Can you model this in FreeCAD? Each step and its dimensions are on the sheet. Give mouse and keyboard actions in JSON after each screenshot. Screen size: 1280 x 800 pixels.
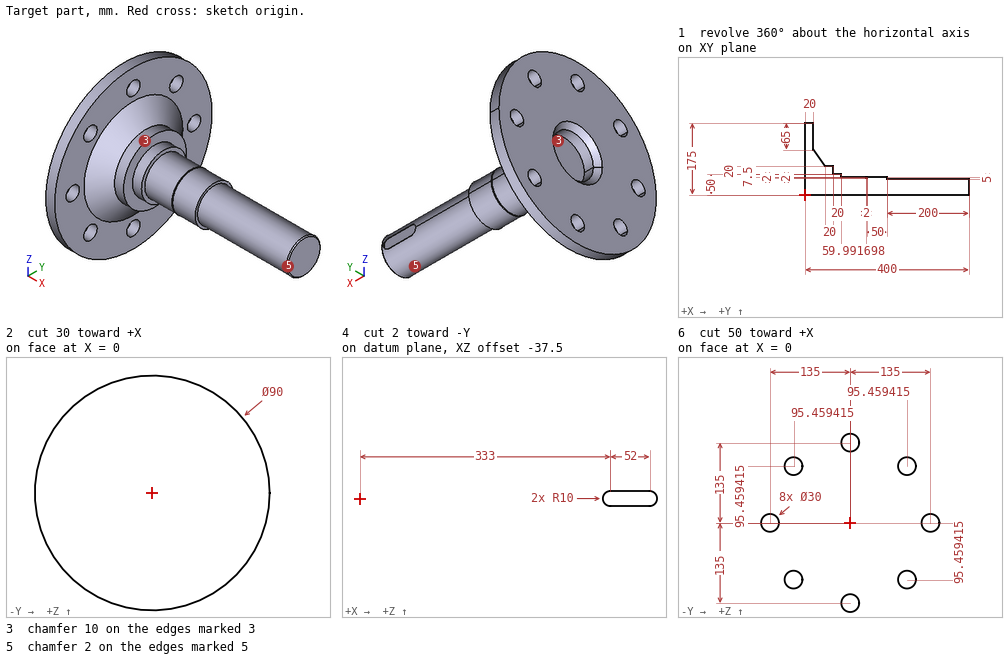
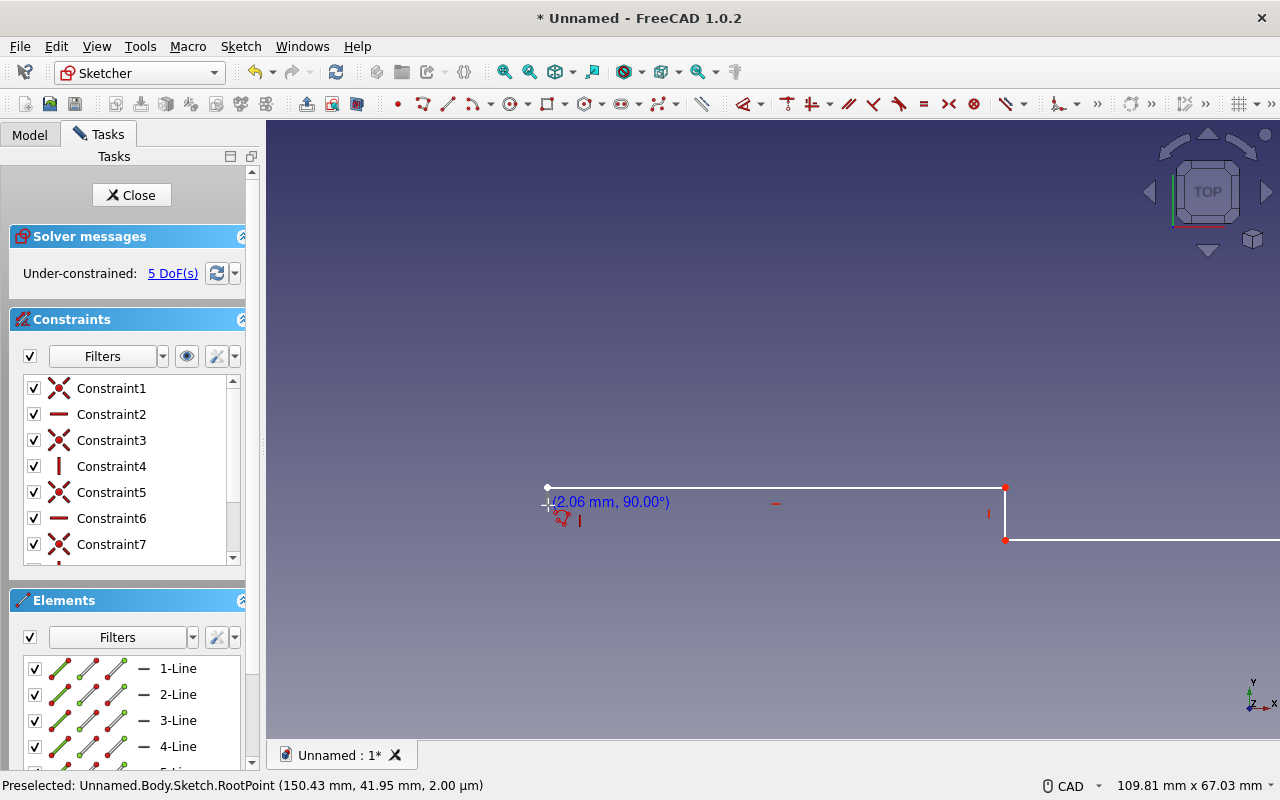
{"action": "left_click", "coordinate": [548, 504]}
{"action": "left_click", "coordinate": [528, 504]}
{"action": "left_click", "coordinate": [528, 485]}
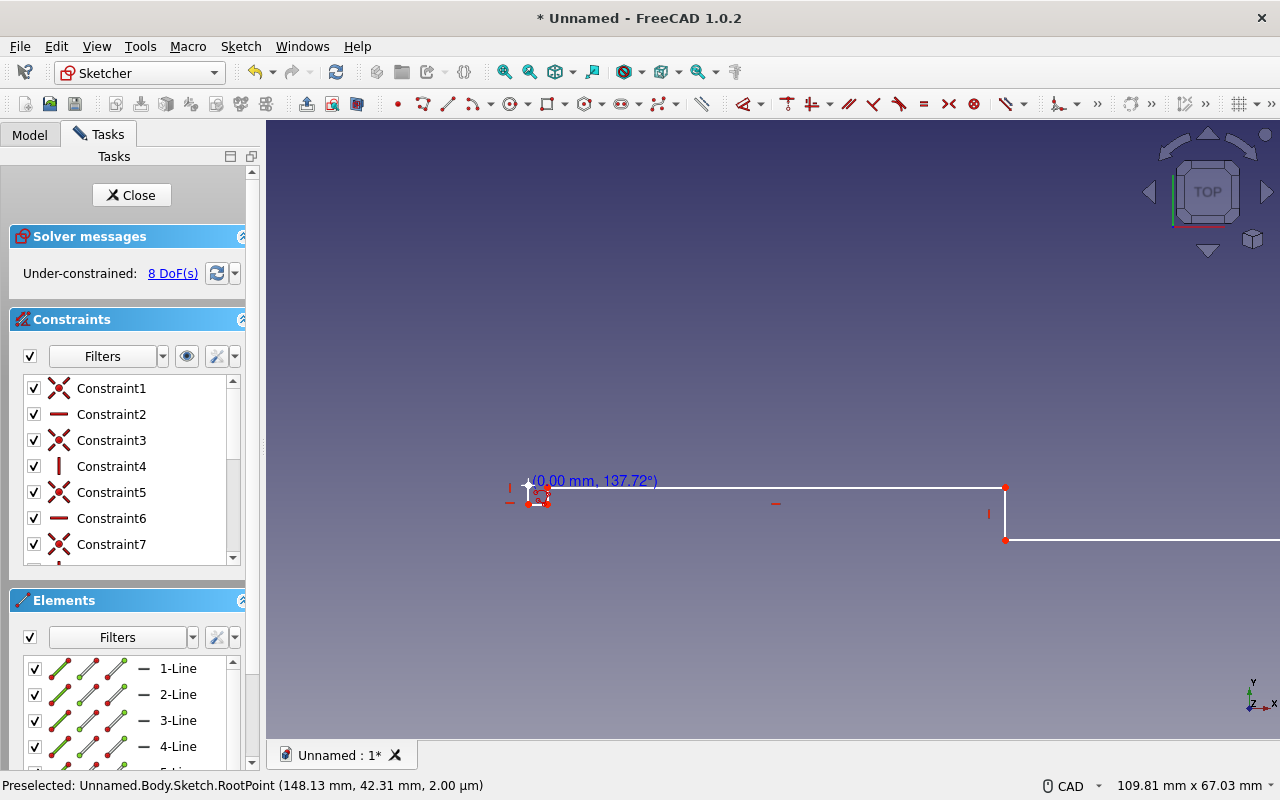
{"action": "scroll", "coordinate": [644, 501], "scroll_direction": "down", "scroll_amount": 9}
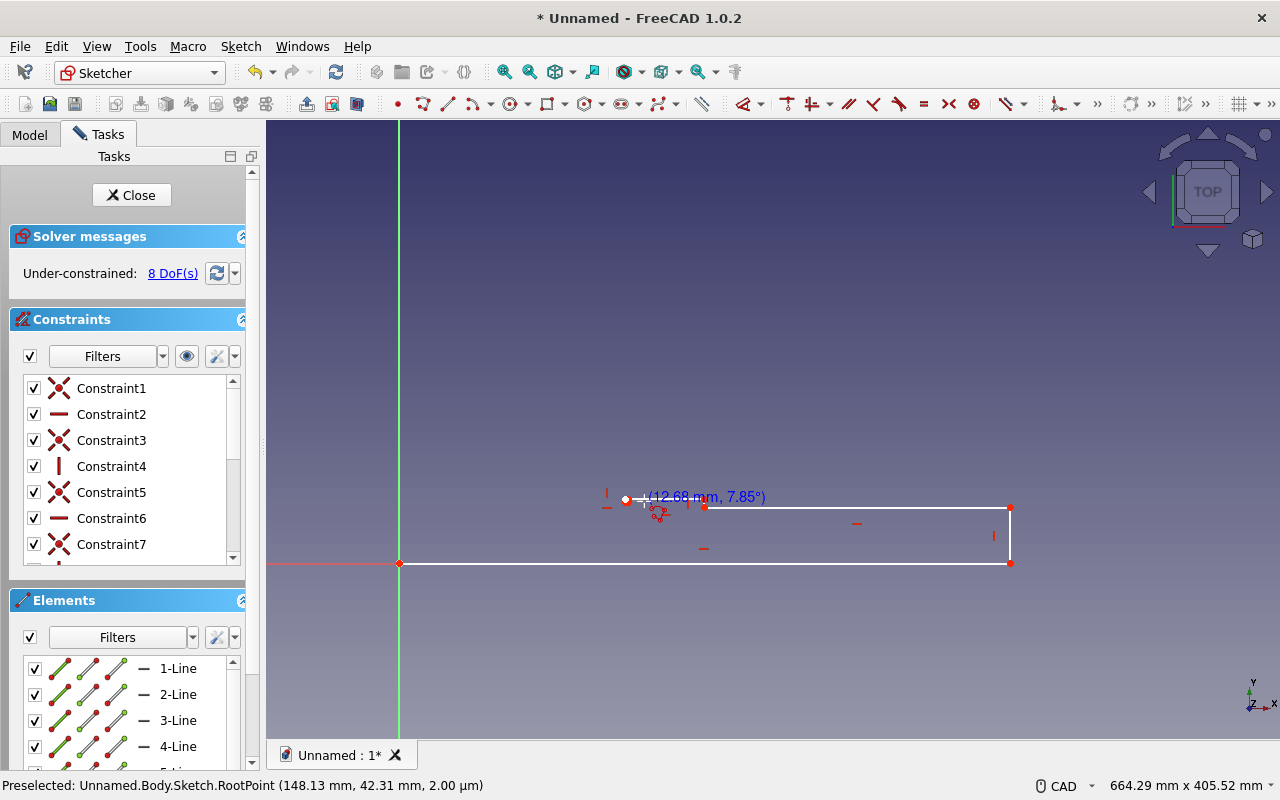
{"action": "left_click", "coordinate": [534, 499]}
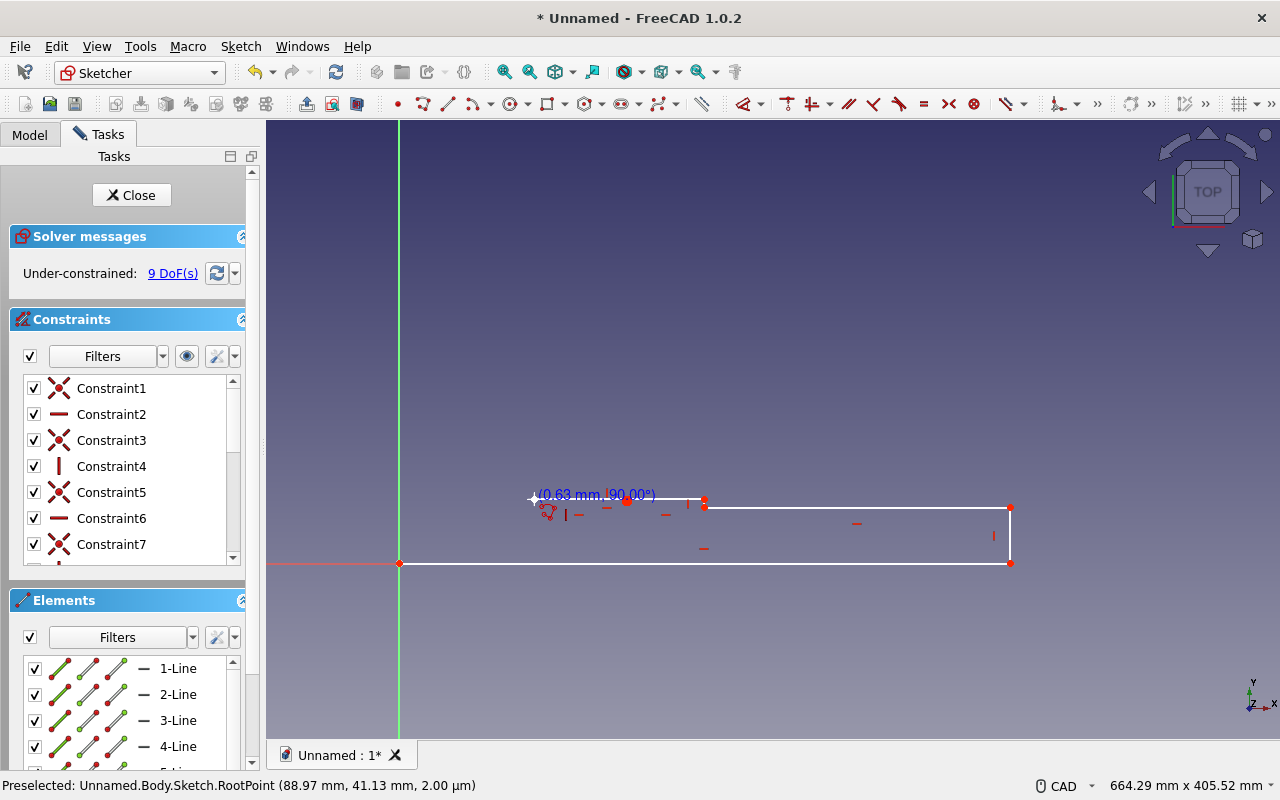
{"action": "scroll", "coordinate": [534, 487], "scroll_direction": "up", "scroll_amount": 2}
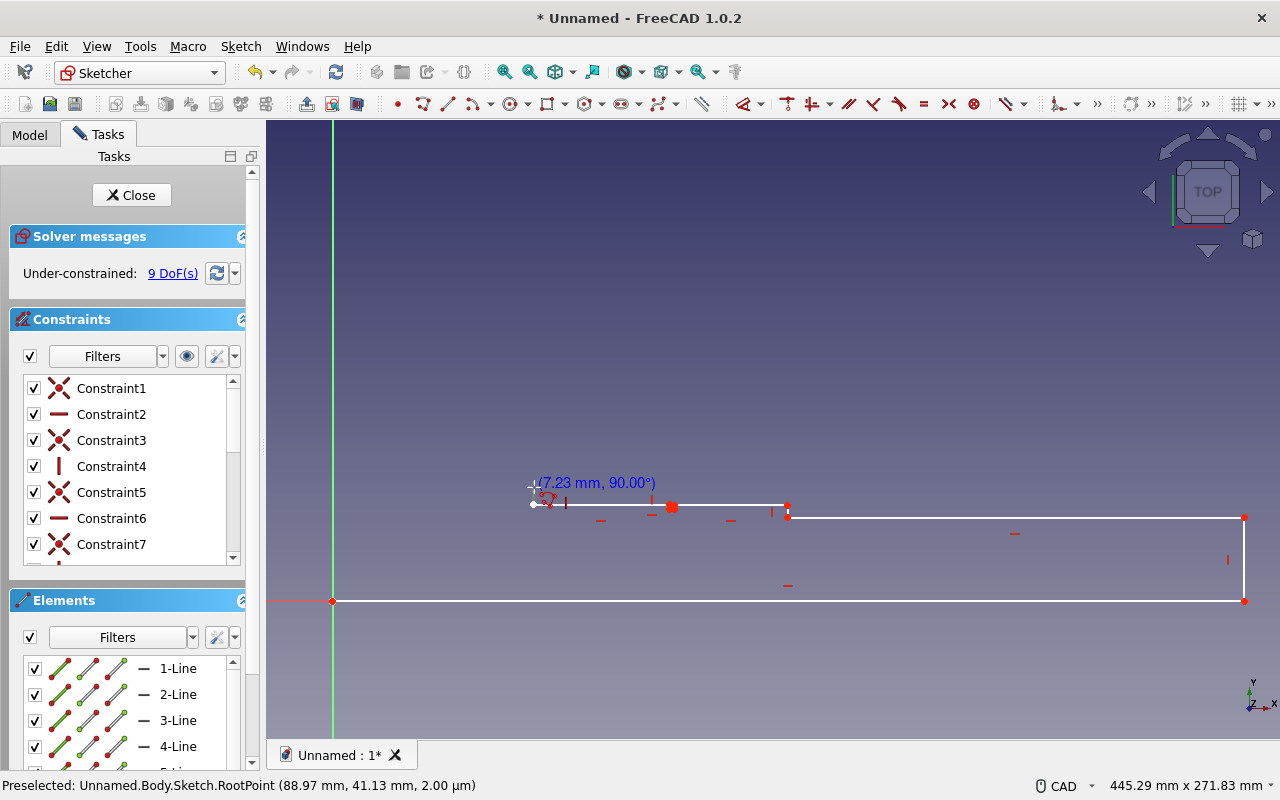
{"action": "left_click", "coordinate": [534, 487]}
{"action": "left_click", "coordinate": [488, 487]}
{"action": "left_click", "coordinate": [488, 442]}
{"action": "left_click", "coordinate": [442, 442]}
{"action": "left_click", "coordinate": [378, 351]}
{"action": "left_click", "coordinate": [378, 203]}
{"action": "left_click", "coordinate": [342, 203]}
{"action": "left_click", "coordinate": [333, 601]}
{"action": "key", "text": "Escape"}
{"action": "key", "text": "Escape"}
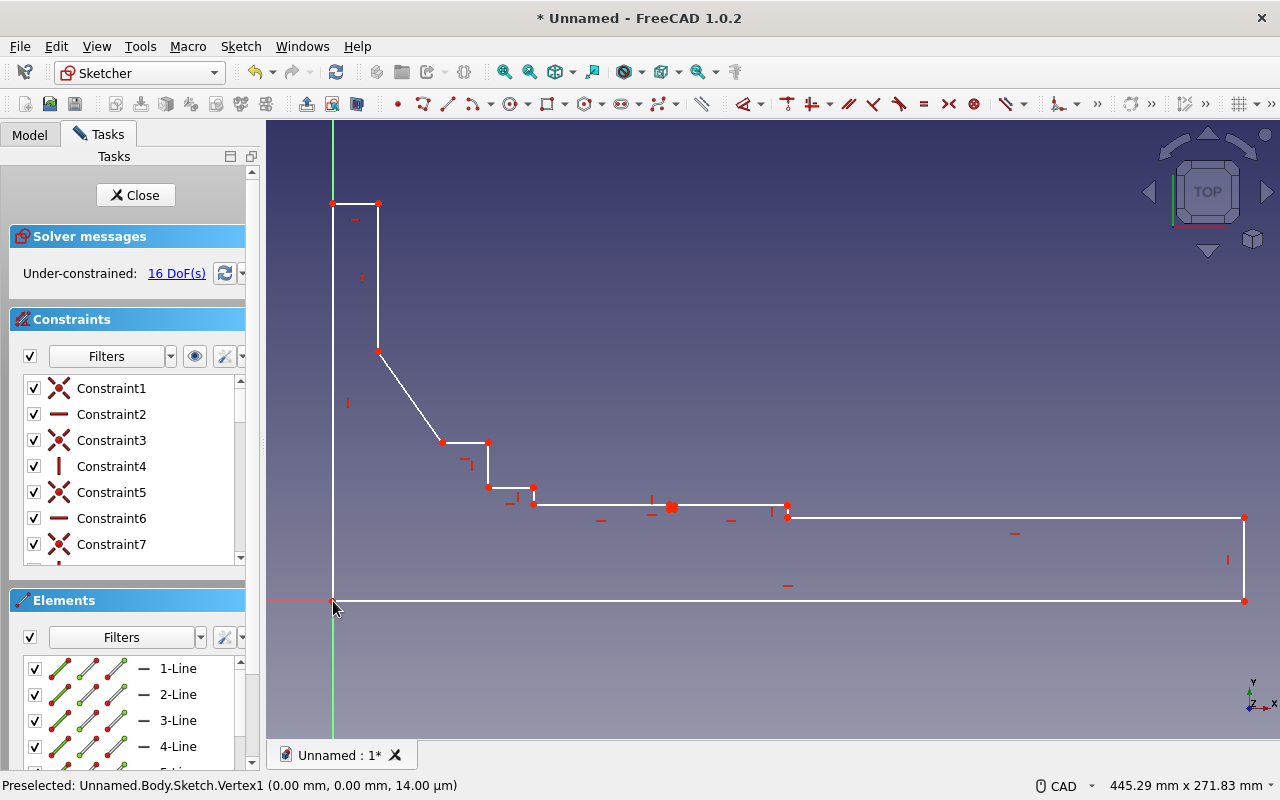
{"action": "left_click", "coordinate": [742, 104]}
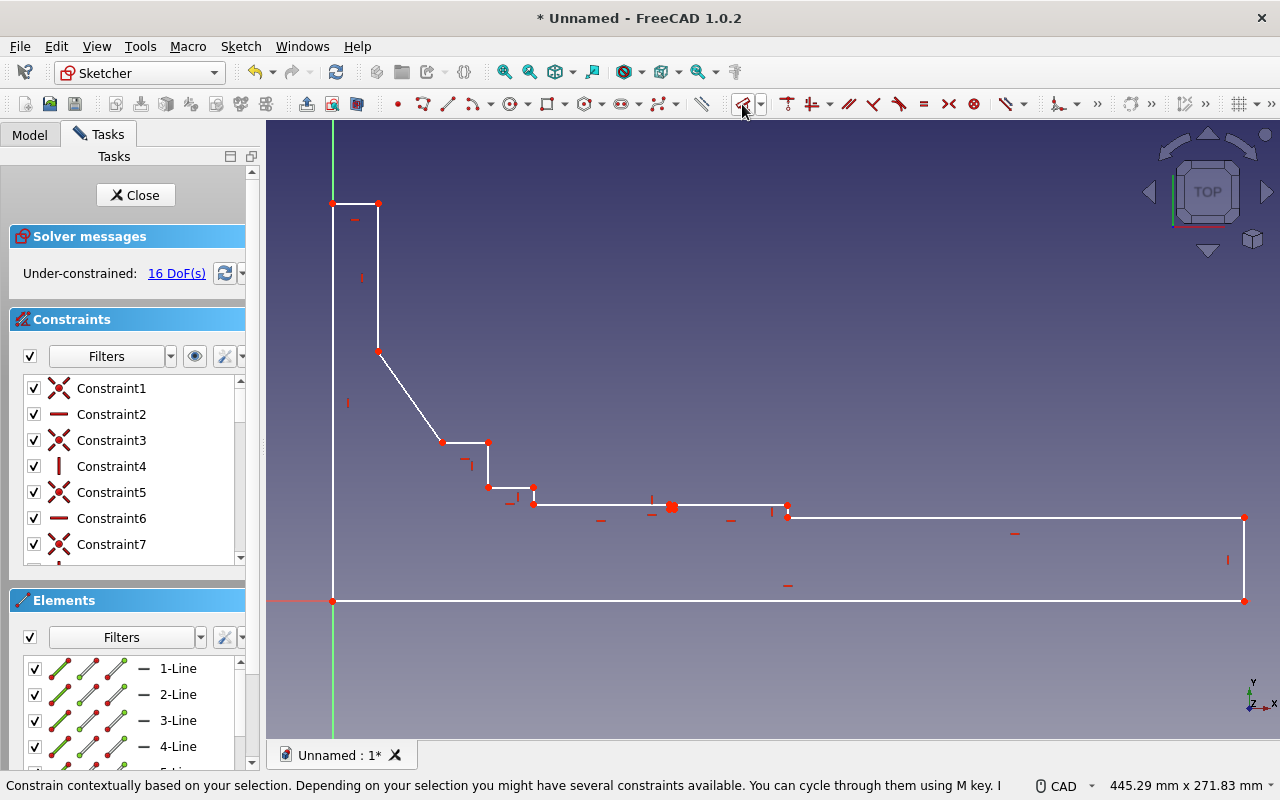
{"action": "scroll", "coordinate": [788, 512], "scroll_direction": "up", "scroll_amount": 7}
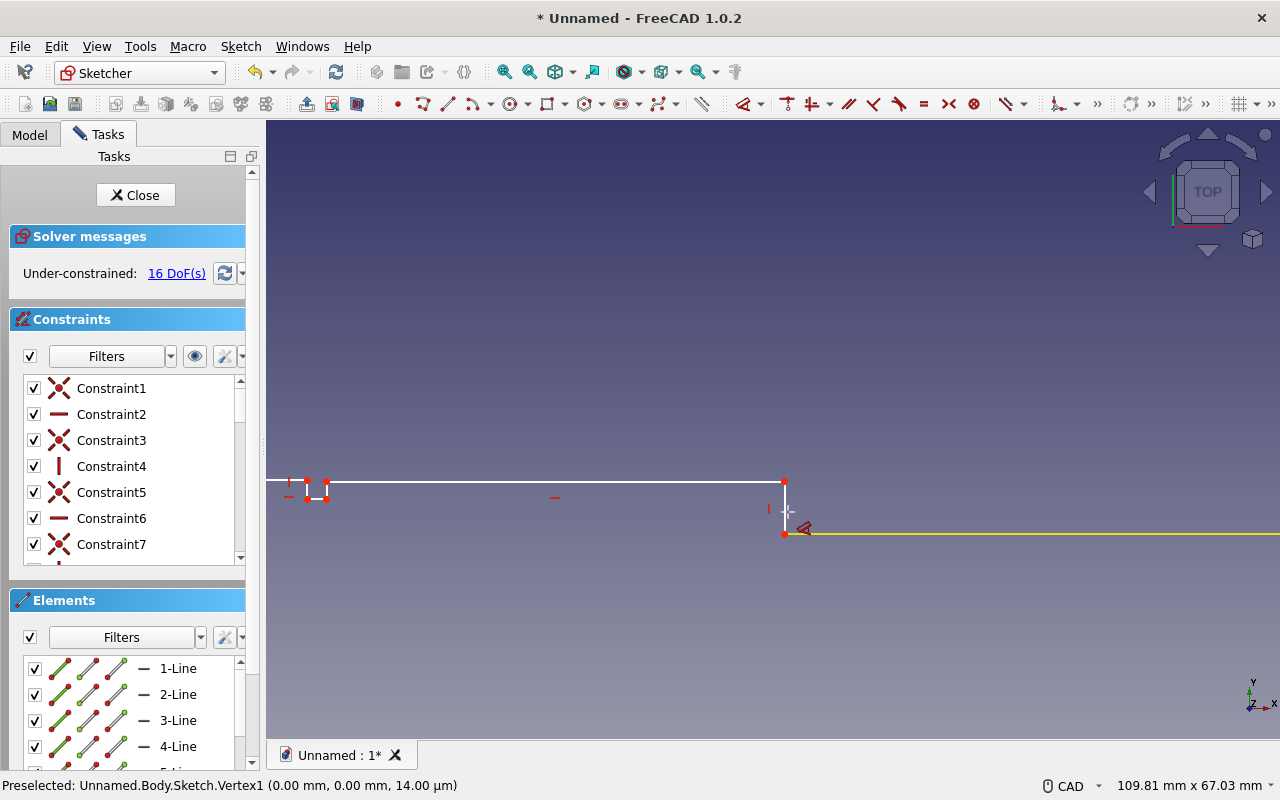
{"action": "left_click", "coordinate": [785, 508]}
{"action": "left_click", "coordinate": [751, 508]}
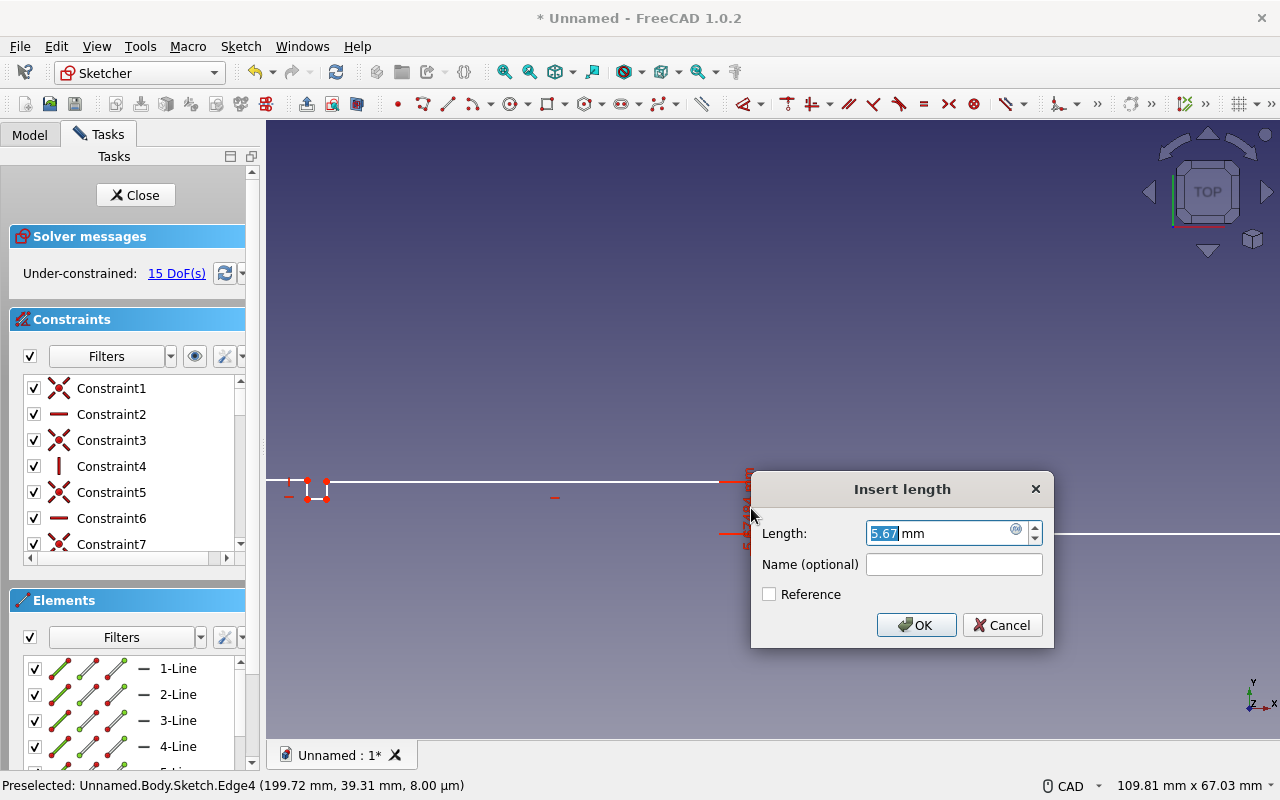
{"action": "type", "text": "5"}
{"action": "key", "text": "Return"}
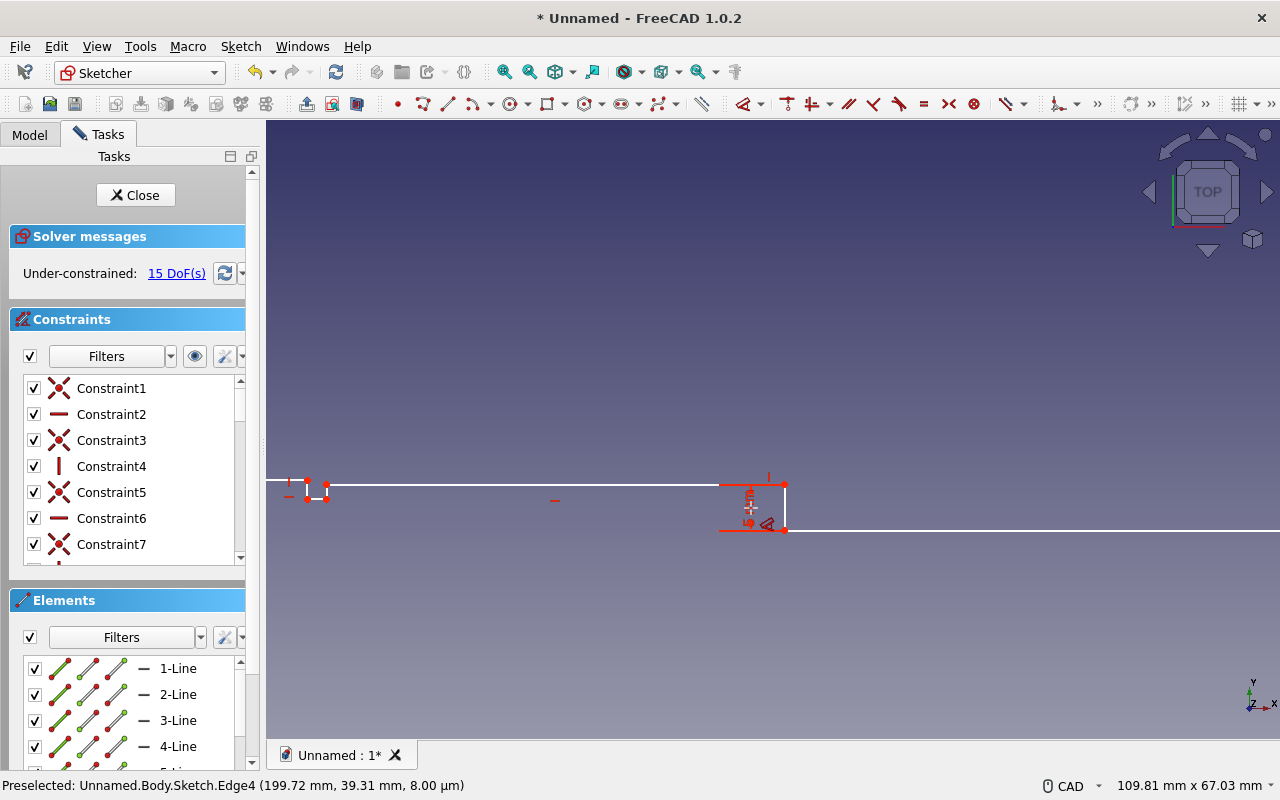
{"action": "scroll", "coordinate": [327, 492], "scroll_direction": "up", "scroll_amount": 4}